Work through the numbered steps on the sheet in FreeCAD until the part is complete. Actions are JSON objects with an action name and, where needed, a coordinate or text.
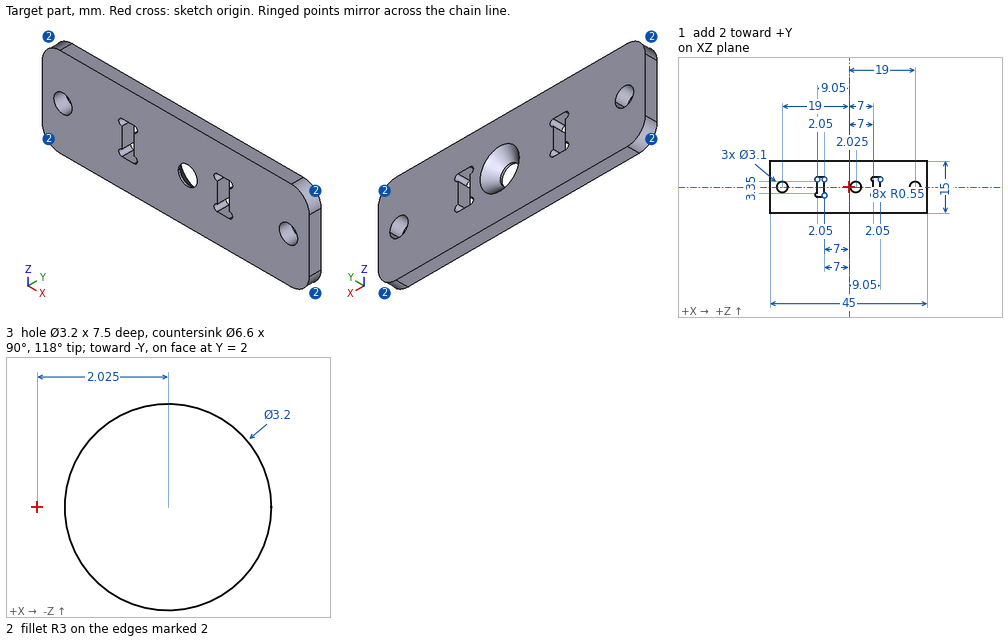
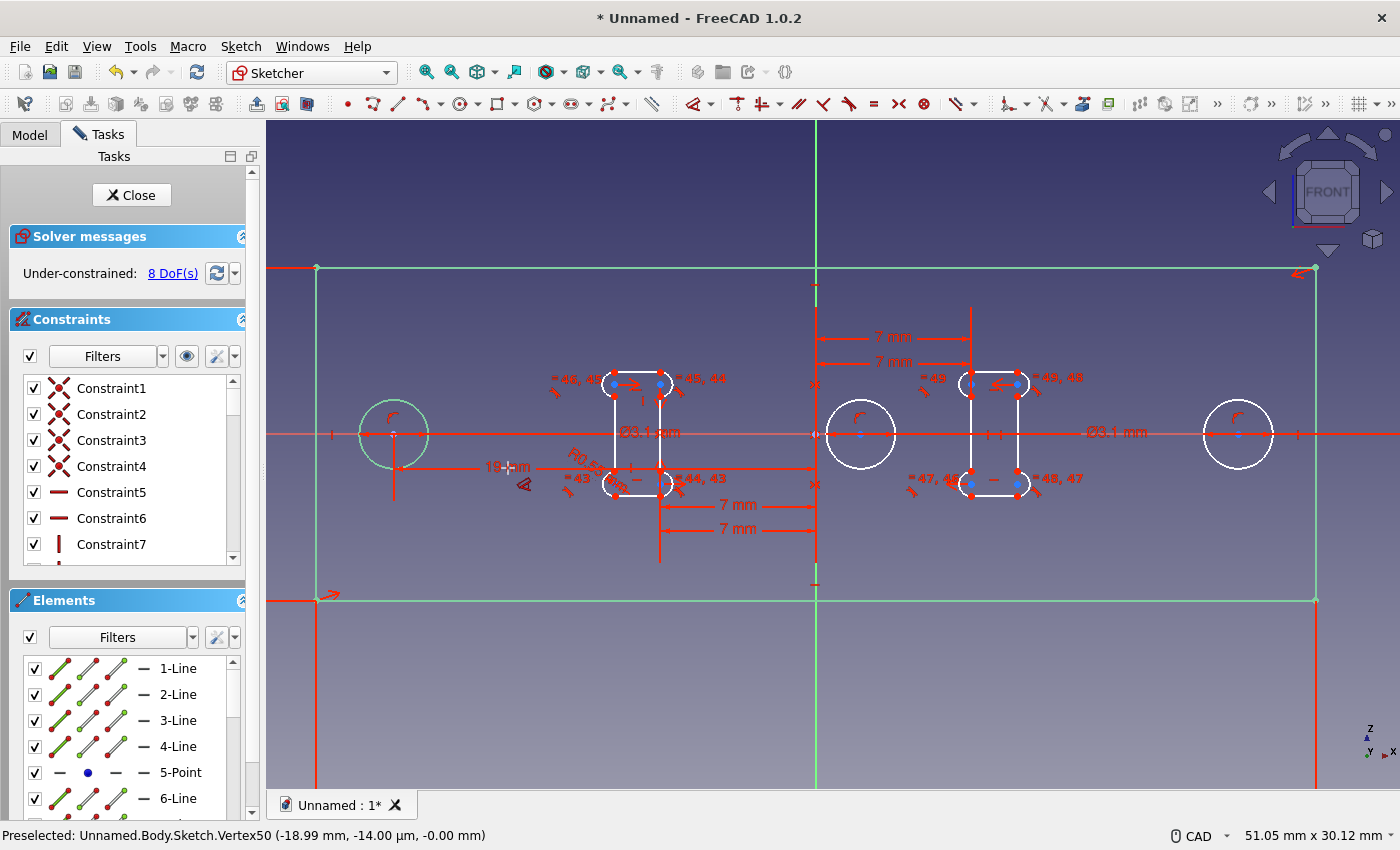
{"action": "scroll", "coordinate": [660, 495], "scroll_direction": "down", "scroll_amount": 2}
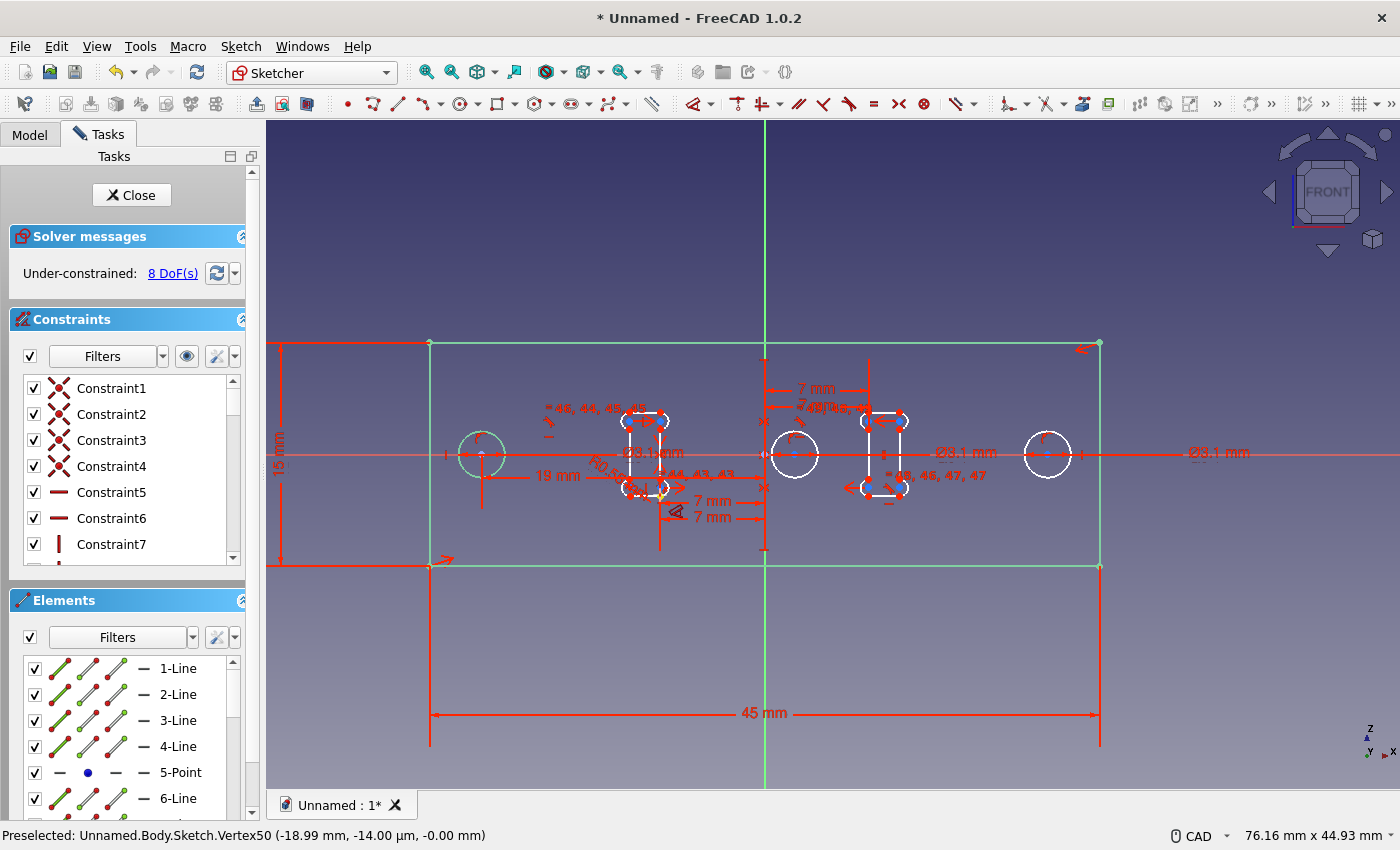
{"action": "left_click", "coordinate": [1048, 455]}
{"action": "left_click", "coordinate": [841, 489]}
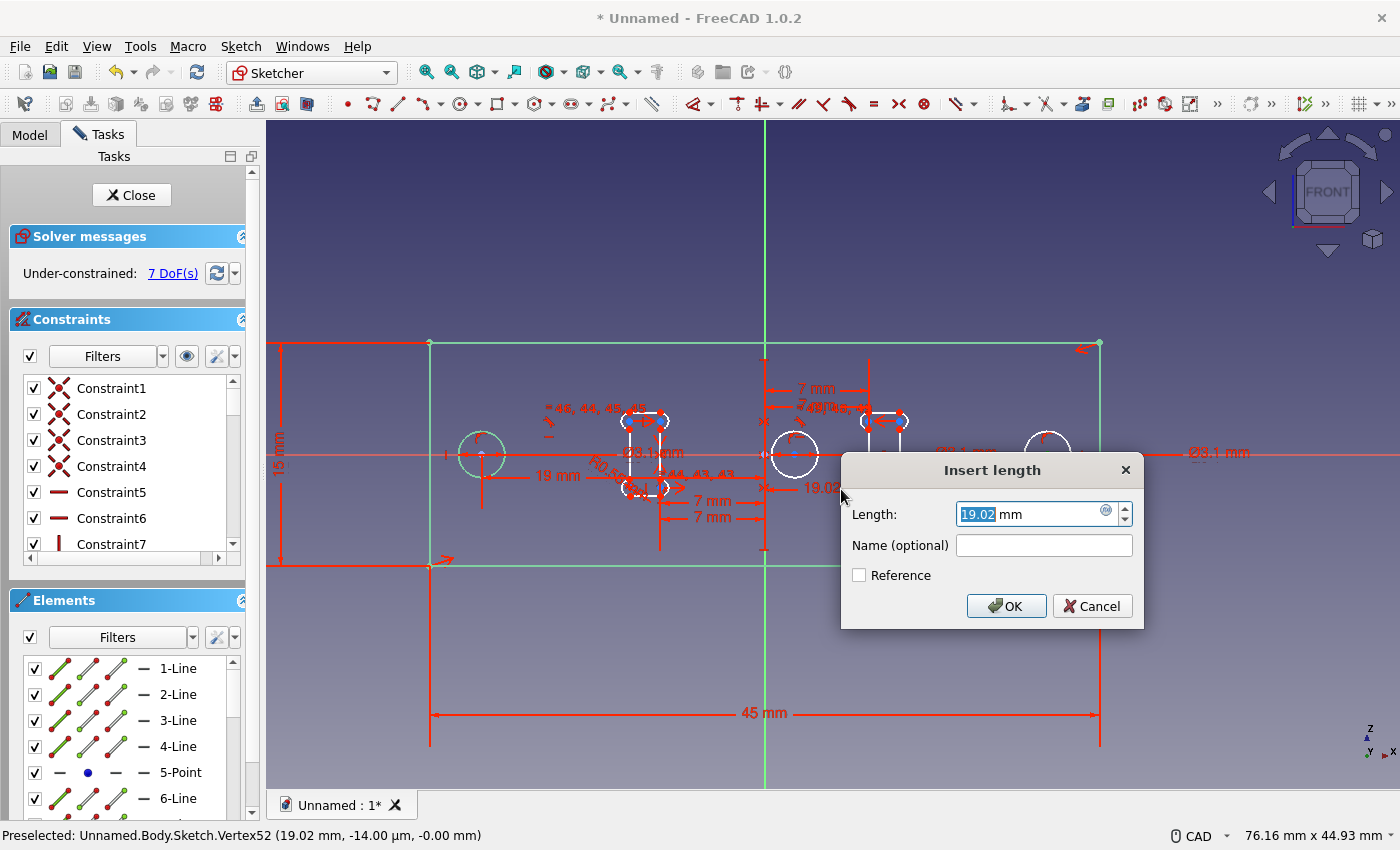
{"action": "type", "text": "19"}
{"action": "key", "text": "Return"}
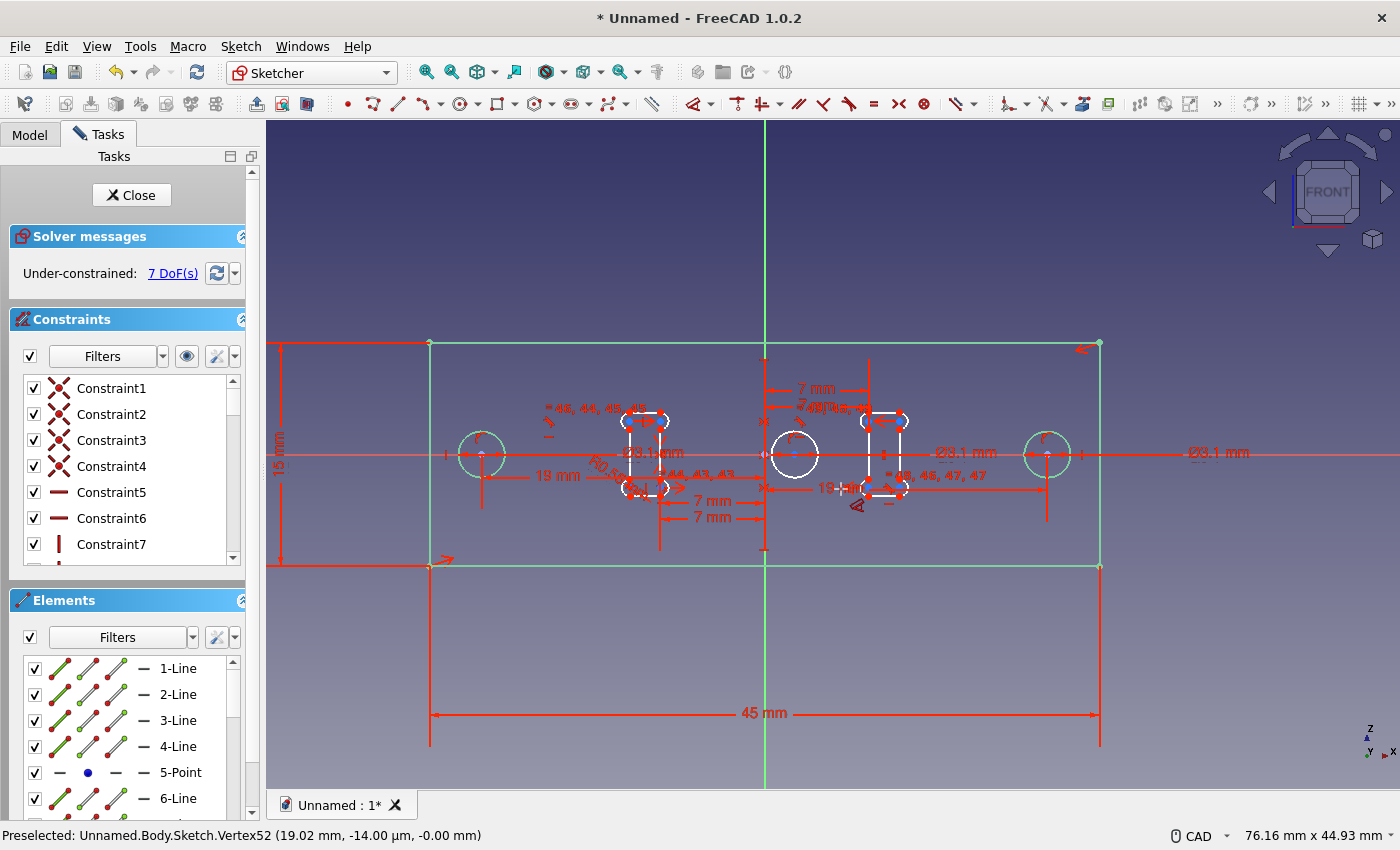
{"action": "scroll", "coordinate": [630, 444], "scroll_direction": "up", "scroll_amount": 2}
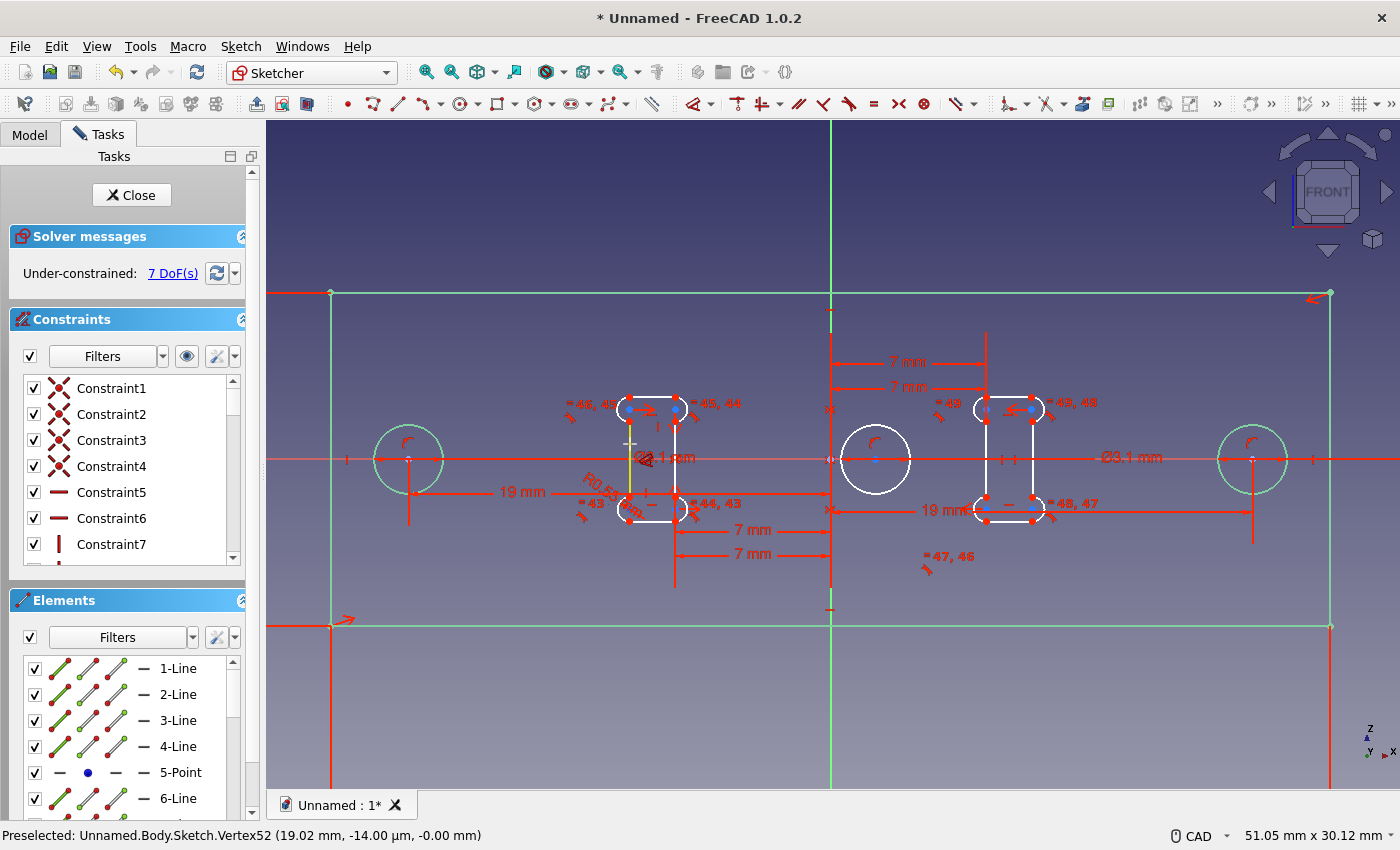
{"action": "left_click", "coordinate": [630, 444]}
{"action": "left_click", "coordinate": [596, 442]}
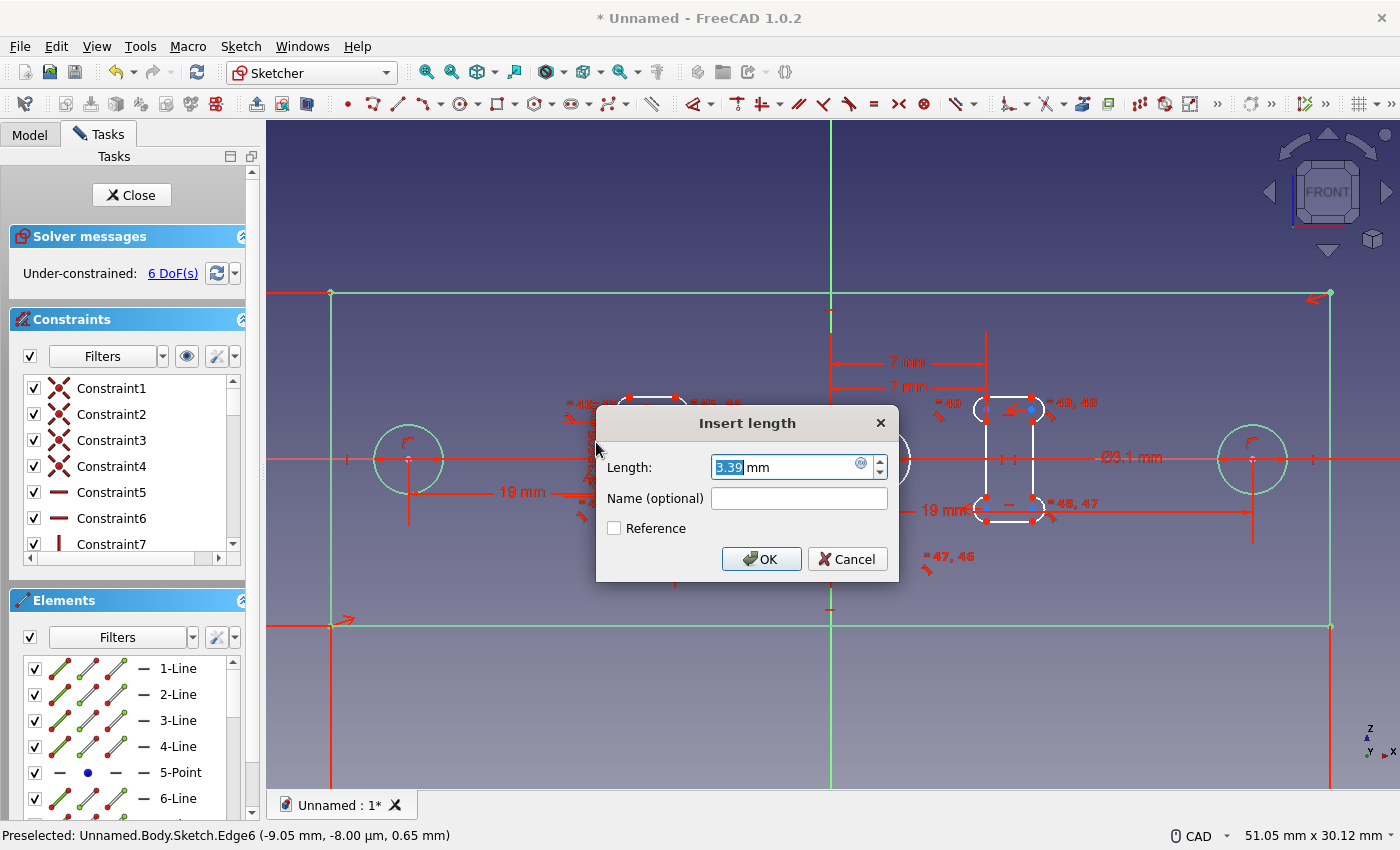
{"action": "type", "text": "3.35"}
{"action": "key", "text": "Return"}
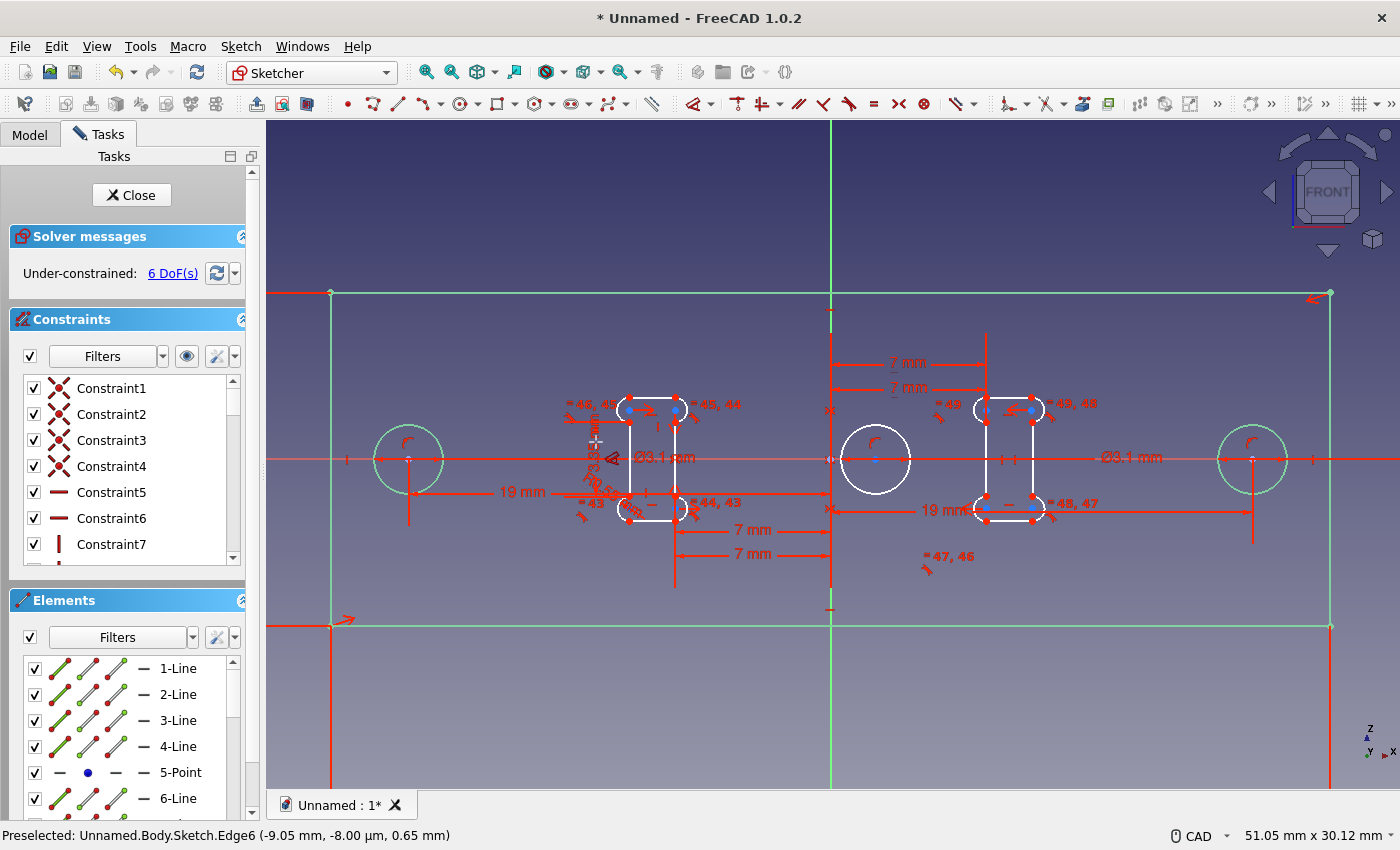
{"action": "left_click", "coordinate": [643, 521]}
{"action": "left_click", "coordinate": [653, 555]}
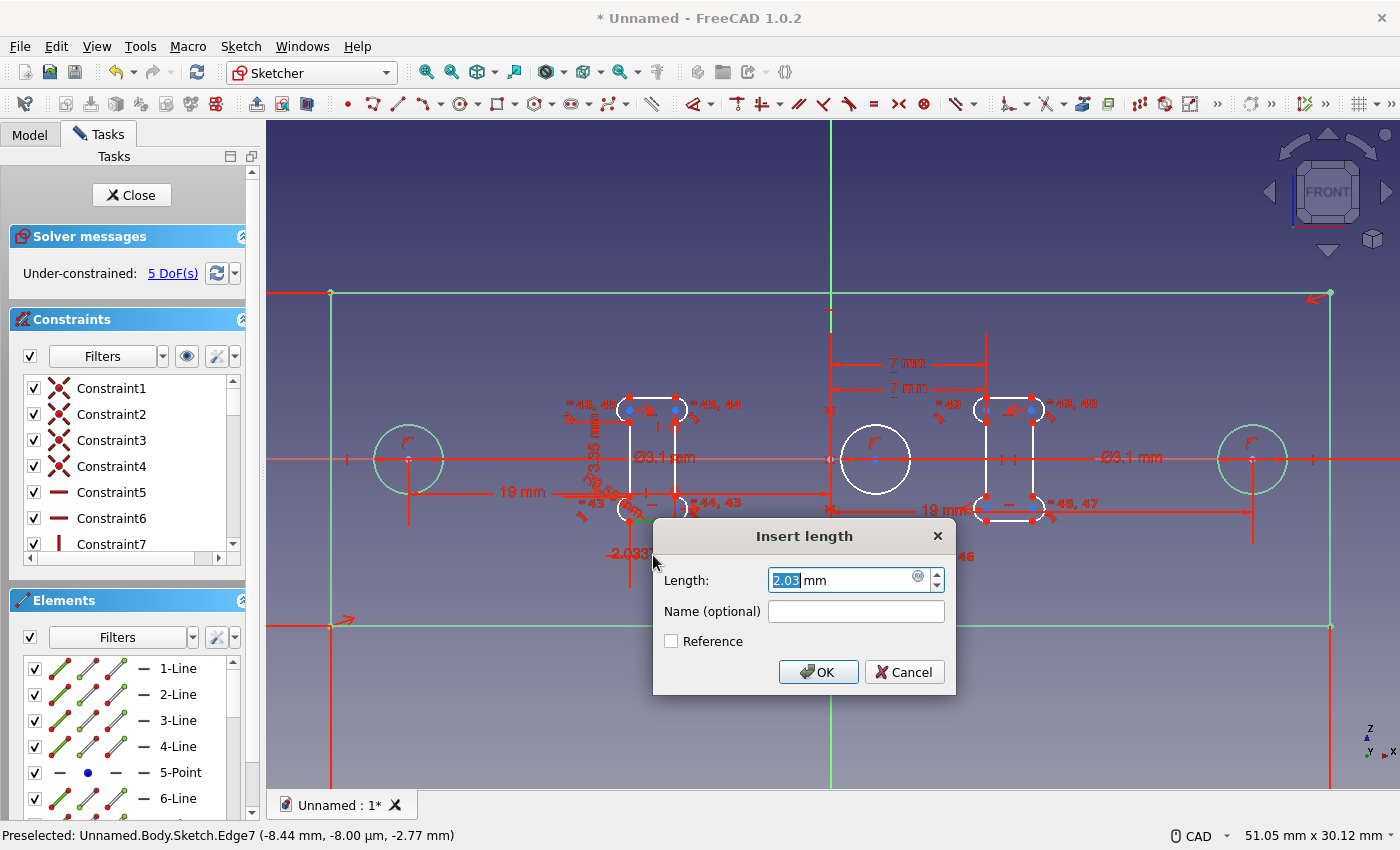
{"action": "type", "text": "2.05"}
{"action": "key", "text": "Return"}